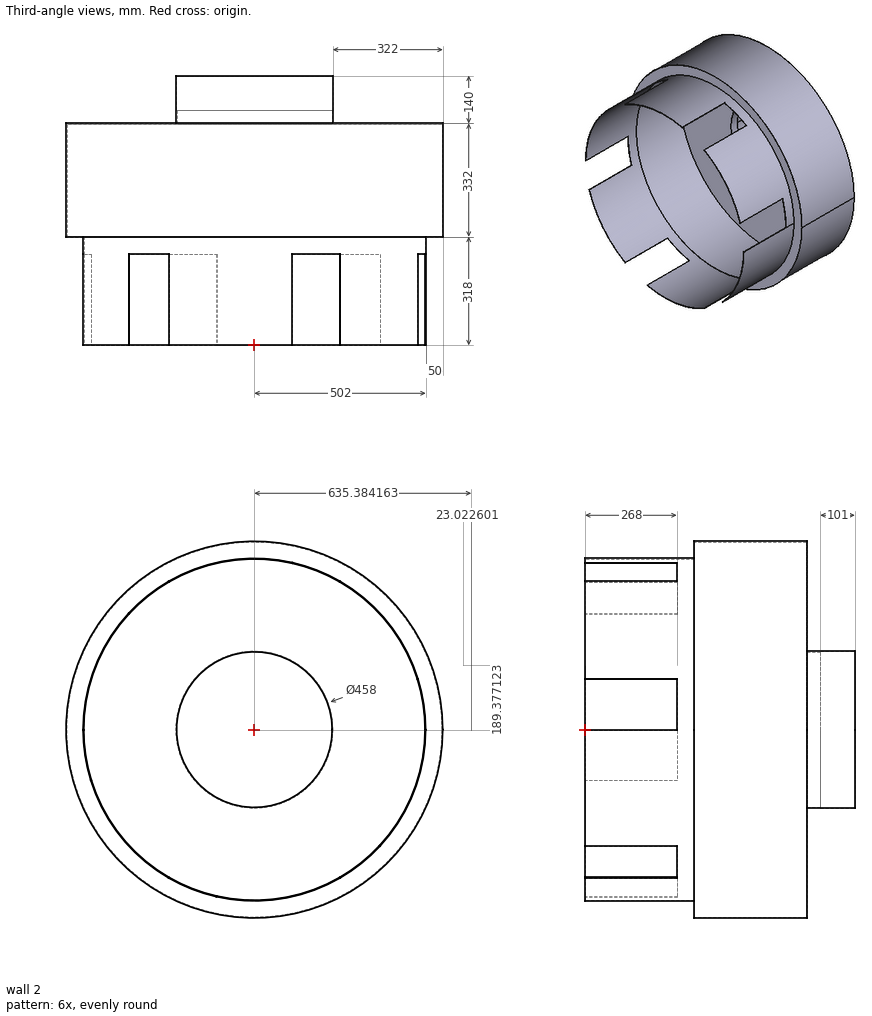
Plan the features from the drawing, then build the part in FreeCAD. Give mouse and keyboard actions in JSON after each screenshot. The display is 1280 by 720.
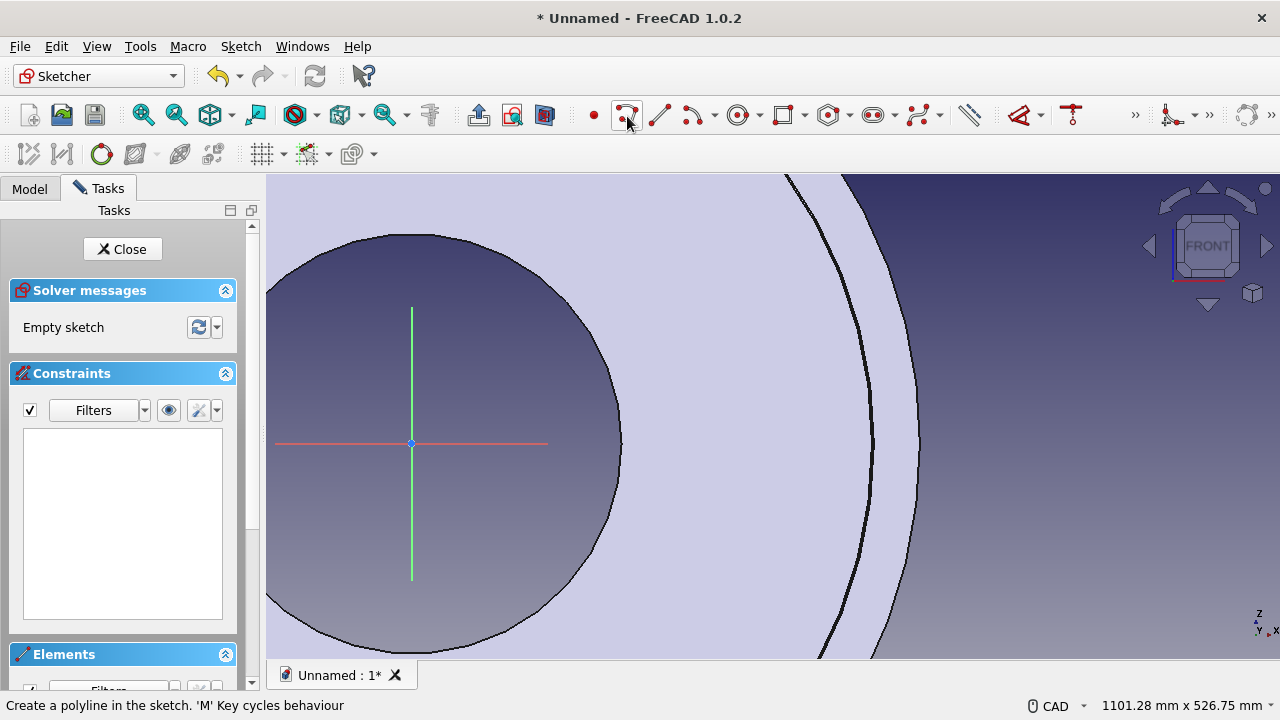
{"action": "left_click", "coordinate": [412, 444]}
{"action": "left_click", "coordinate": [975, 269]}
{"action": "left_click", "coordinate": [997, 435]}
{"action": "left_click", "coordinate": [412, 444]}
{"action": "key", "text": "Escape"}
{"action": "key", "text": "Escape"}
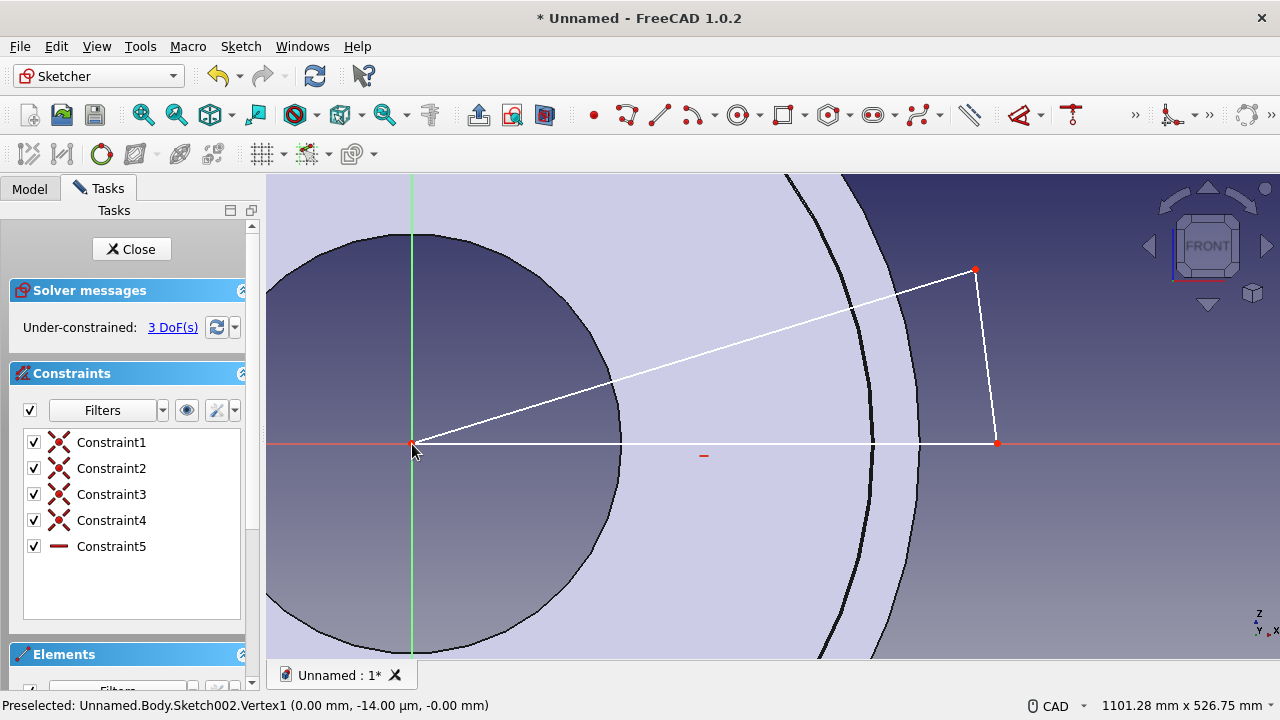
{"action": "left_click", "coordinate": [1018, 116]}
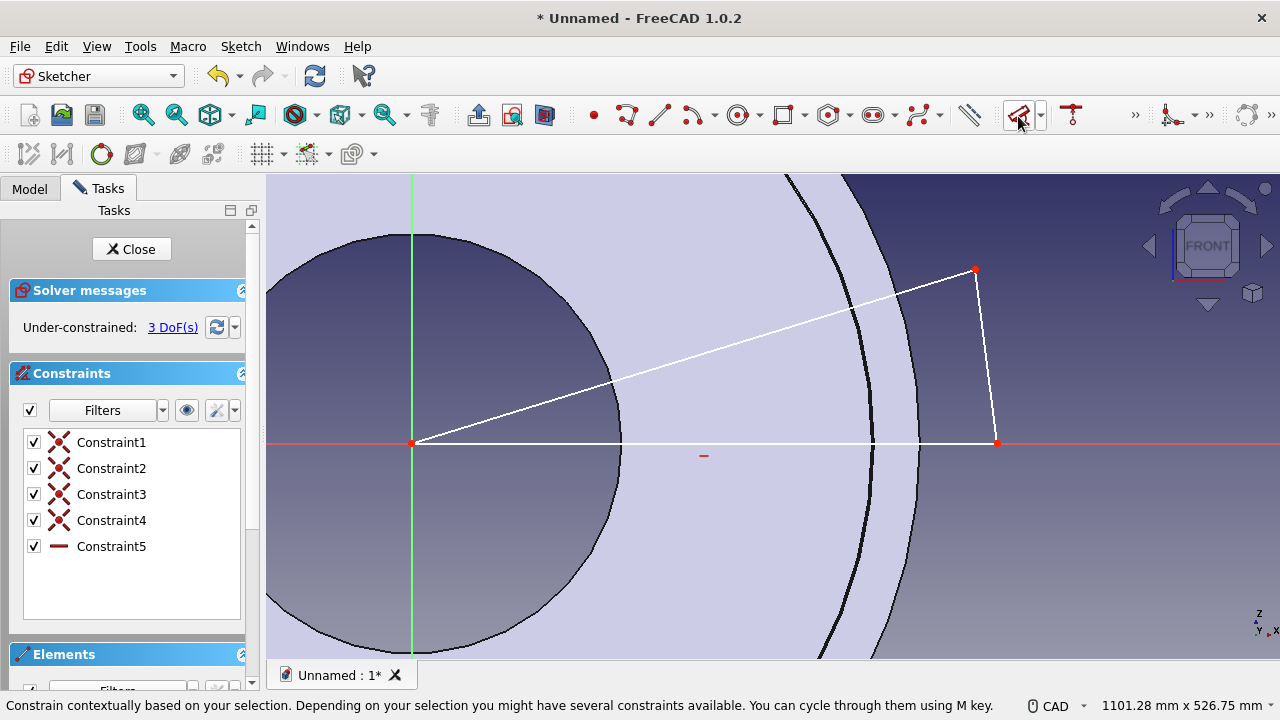
{"action": "left_click", "coordinate": [821, 444]}
{"action": "left_click", "coordinate": [704, 478]}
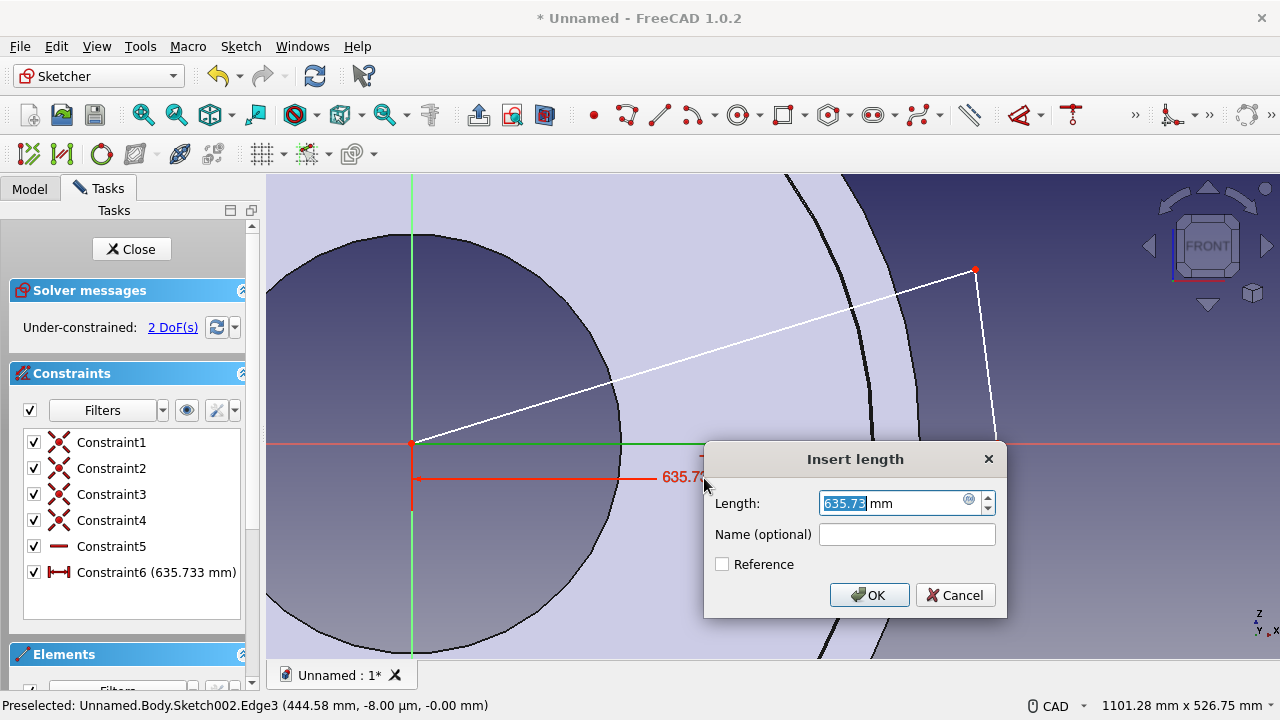
{"action": "type", "text": "635.384163"}
{"action": "key", "text": "Return"}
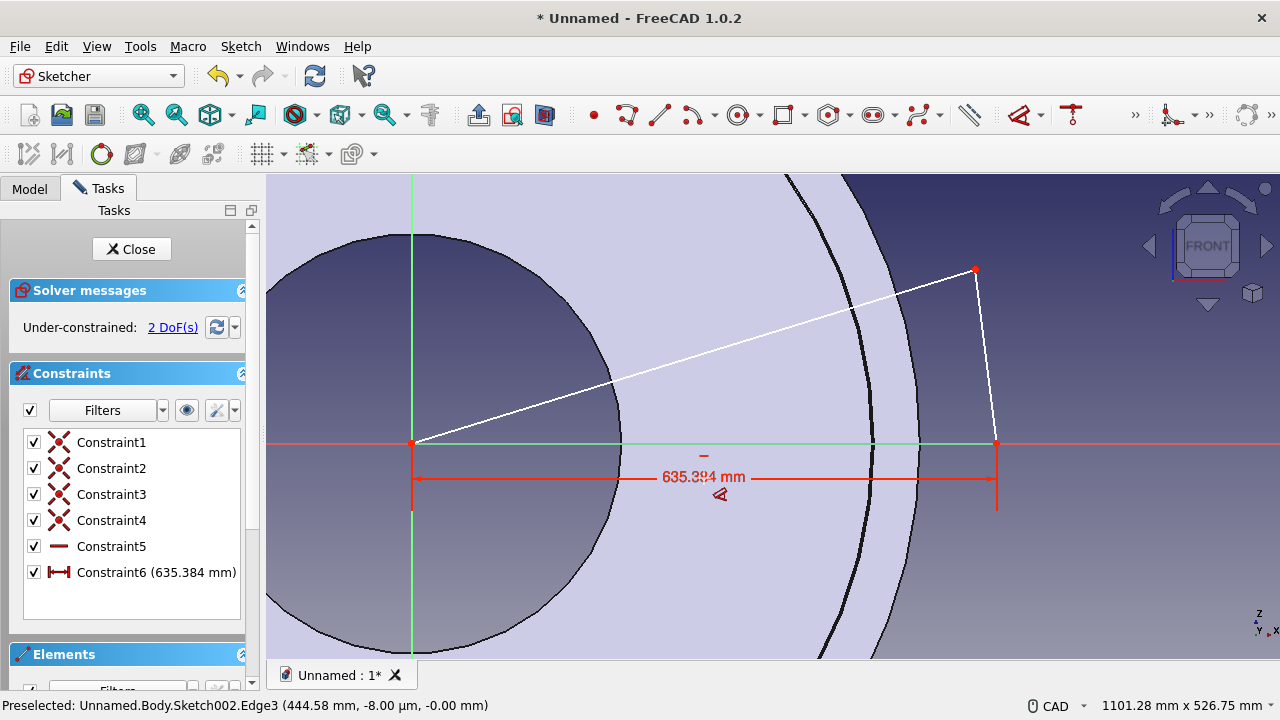
{"action": "scroll", "coordinate": [982, 322], "scroll_direction": "up", "scroll_amount": 4}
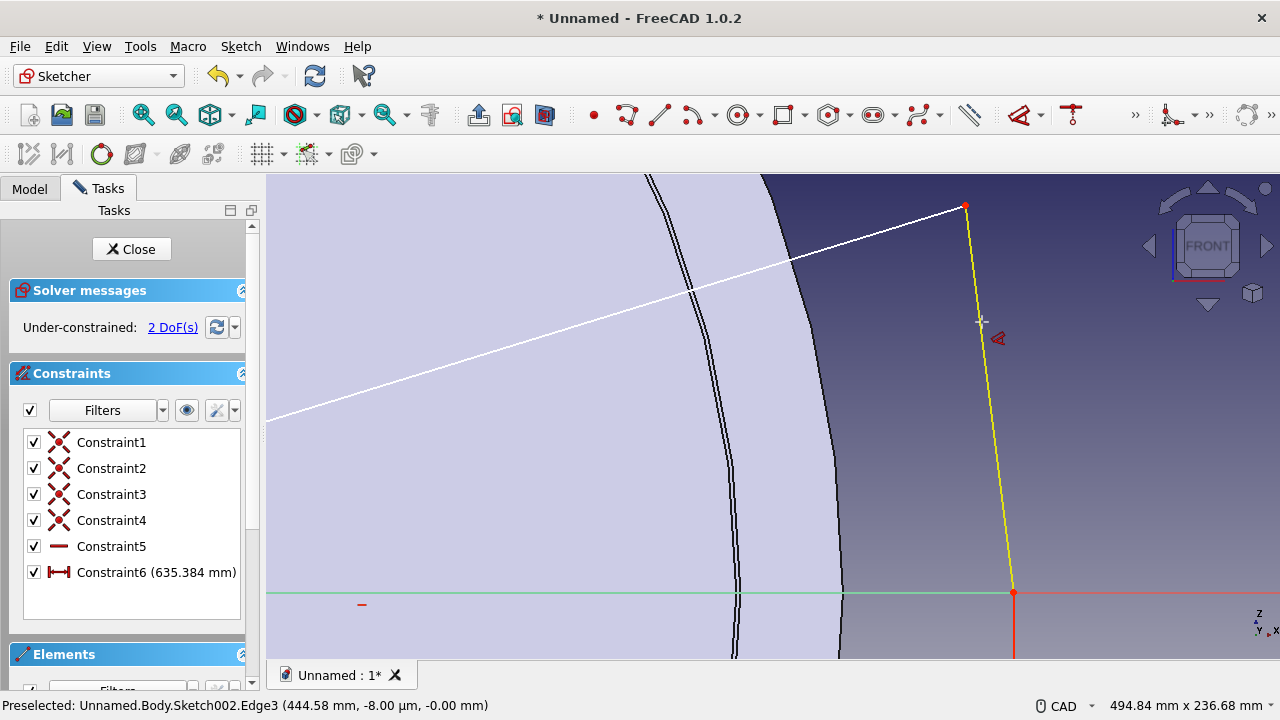
{"action": "left_click", "coordinate": [980, 322]}
{"action": "left_click", "coordinate": [990, 627]}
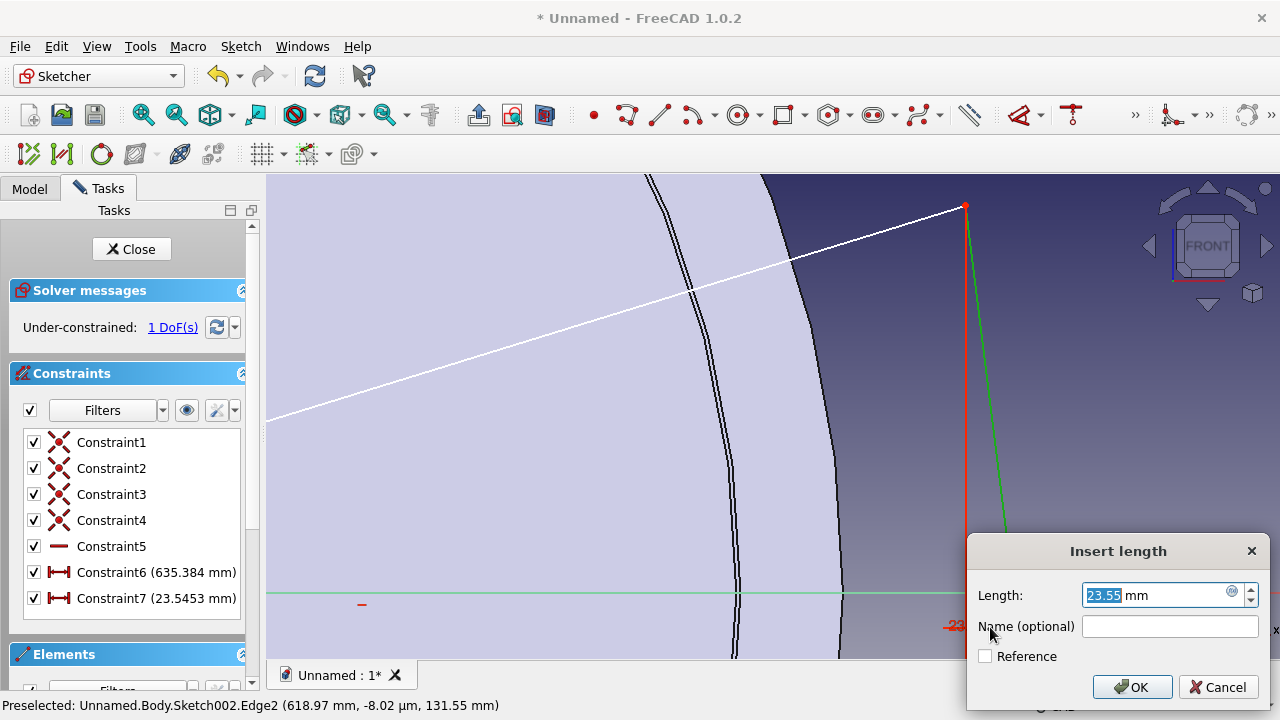
{"action": "type", "text": "23.022601"}
{"action": "key", "text": "Return"}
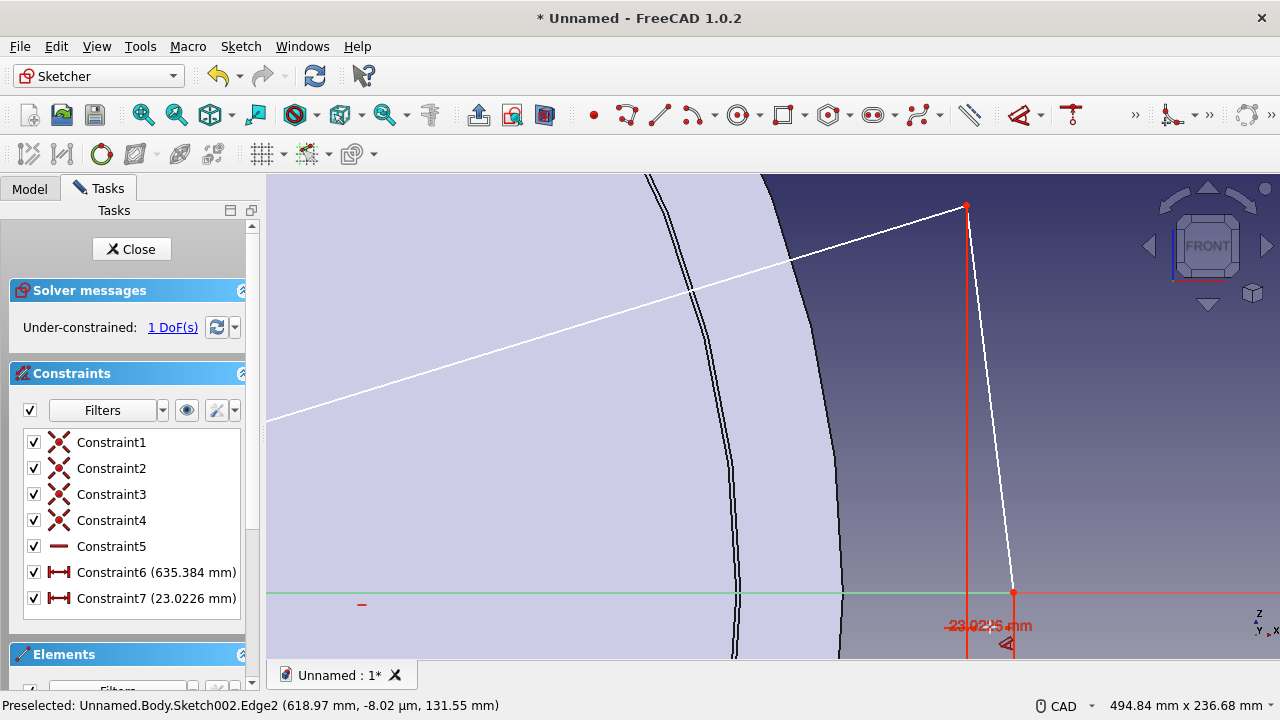
{"action": "left_click", "coordinate": [967, 206]}
{"action": "left_click", "coordinate": [1001, 310]}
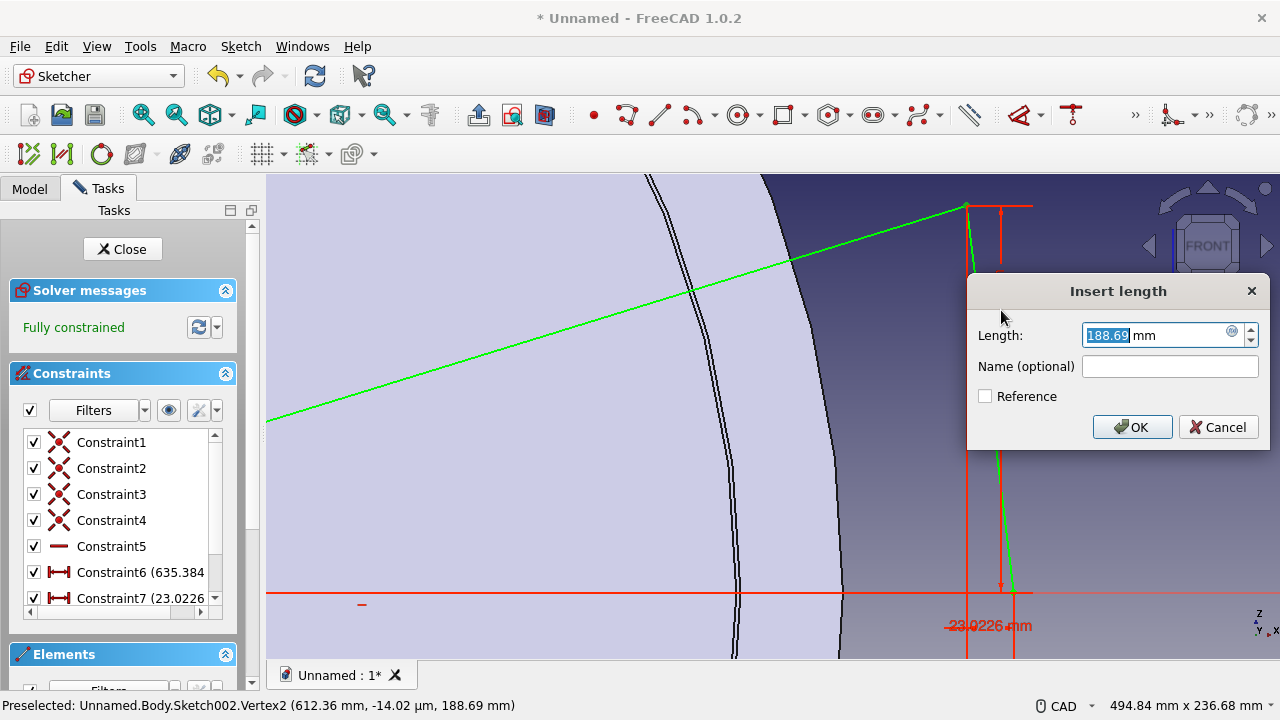
{"action": "type", "text": "189.377123"}
{"action": "key", "text": "Return"}
{"action": "key", "text": "Escape"}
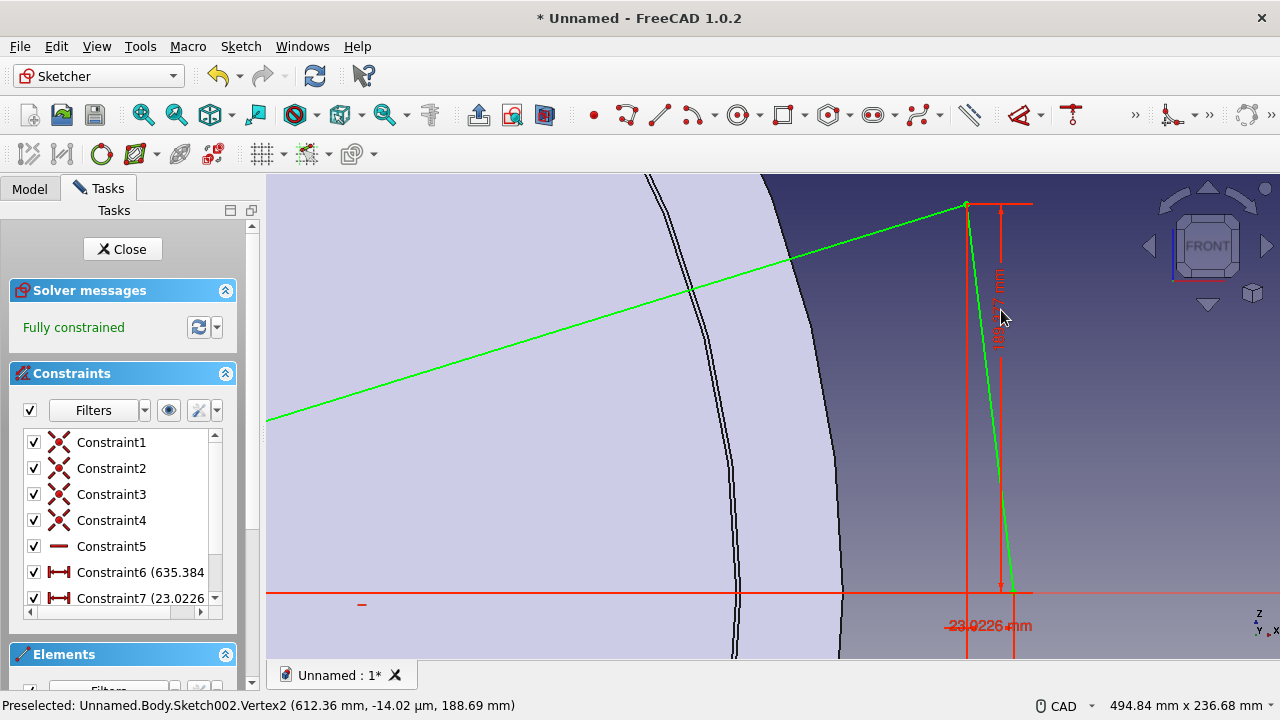
{"action": "left_click", "coordinate": [123, 249]}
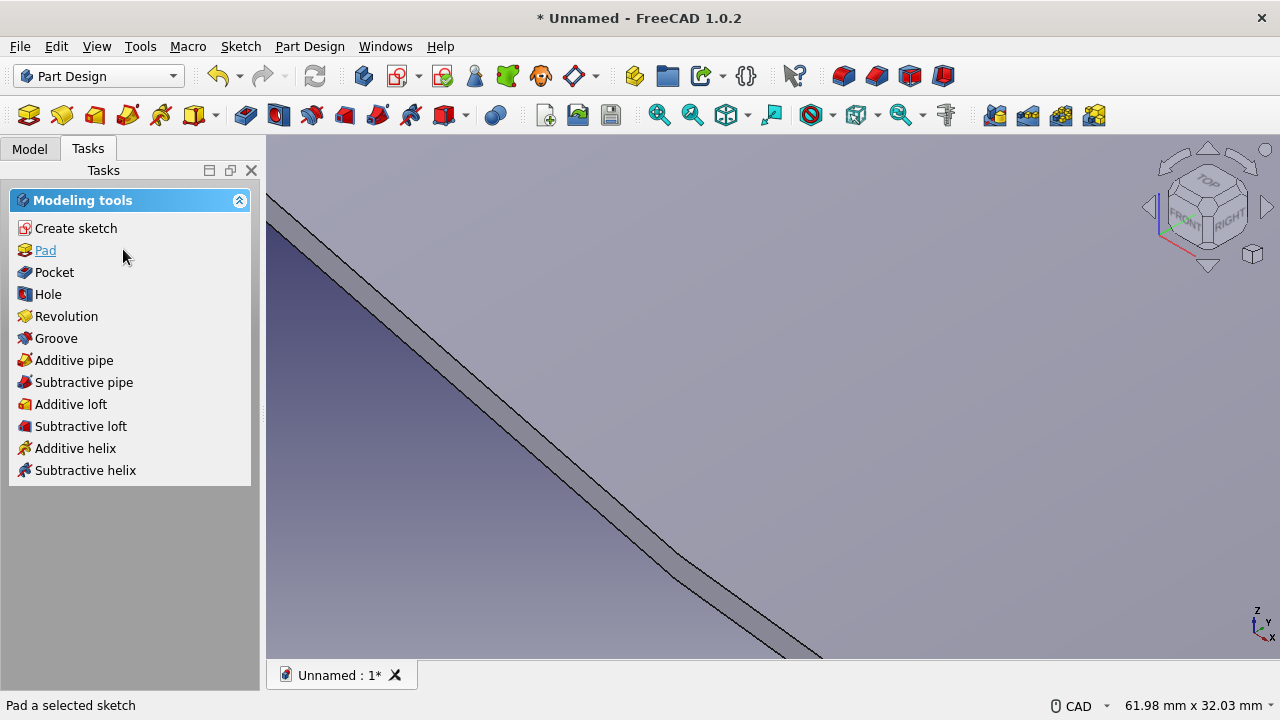
{"action": "left_click", "coordinate": [246, 116]}